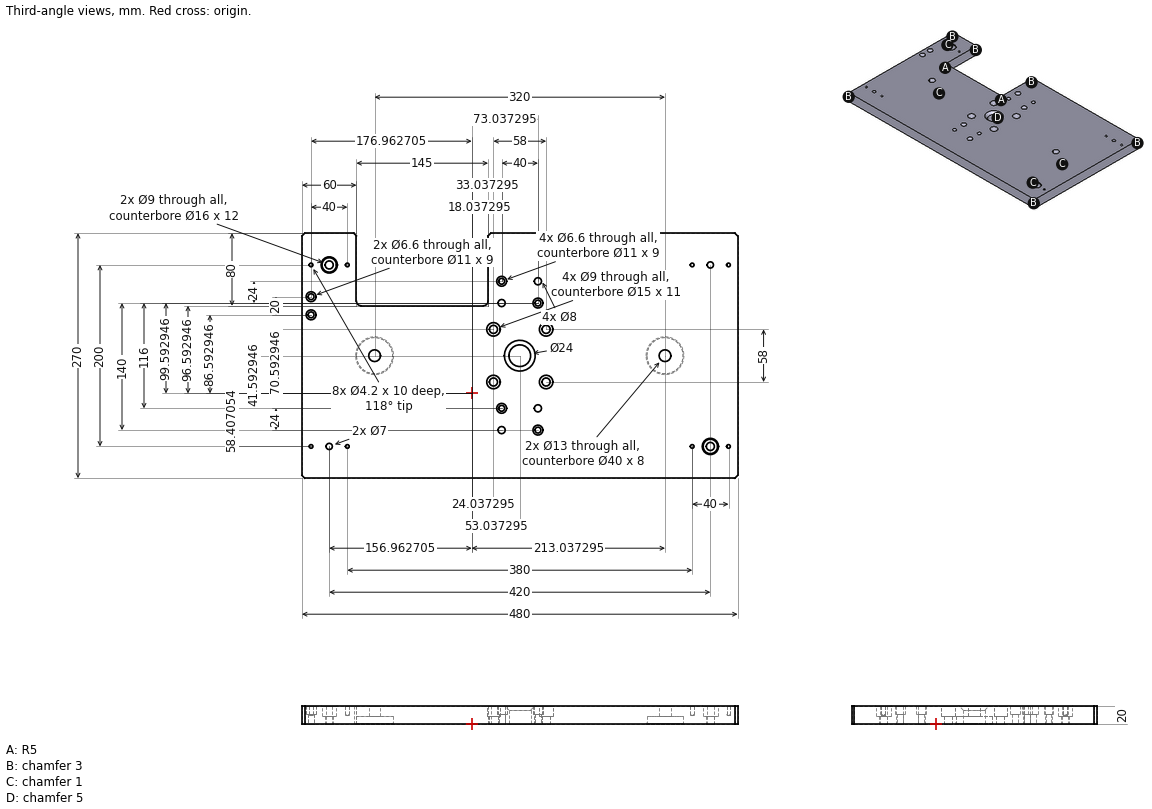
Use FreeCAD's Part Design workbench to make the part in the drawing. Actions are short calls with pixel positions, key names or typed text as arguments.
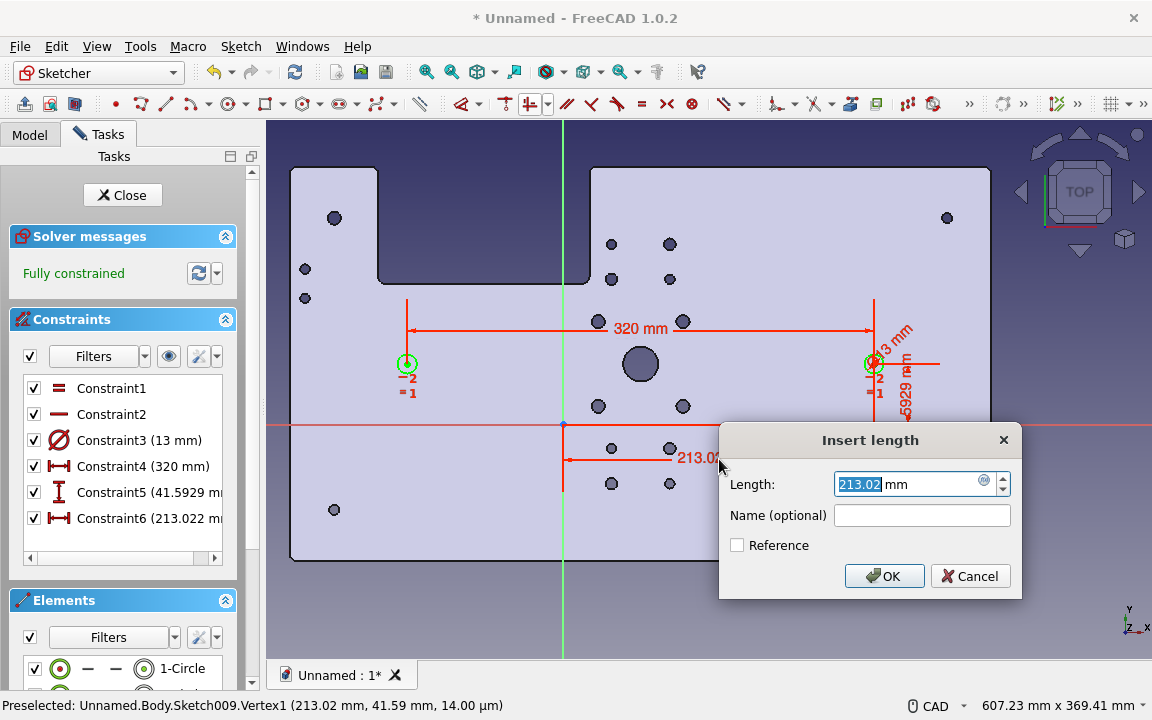
text(213.037295)
key(Return)
key(Escape)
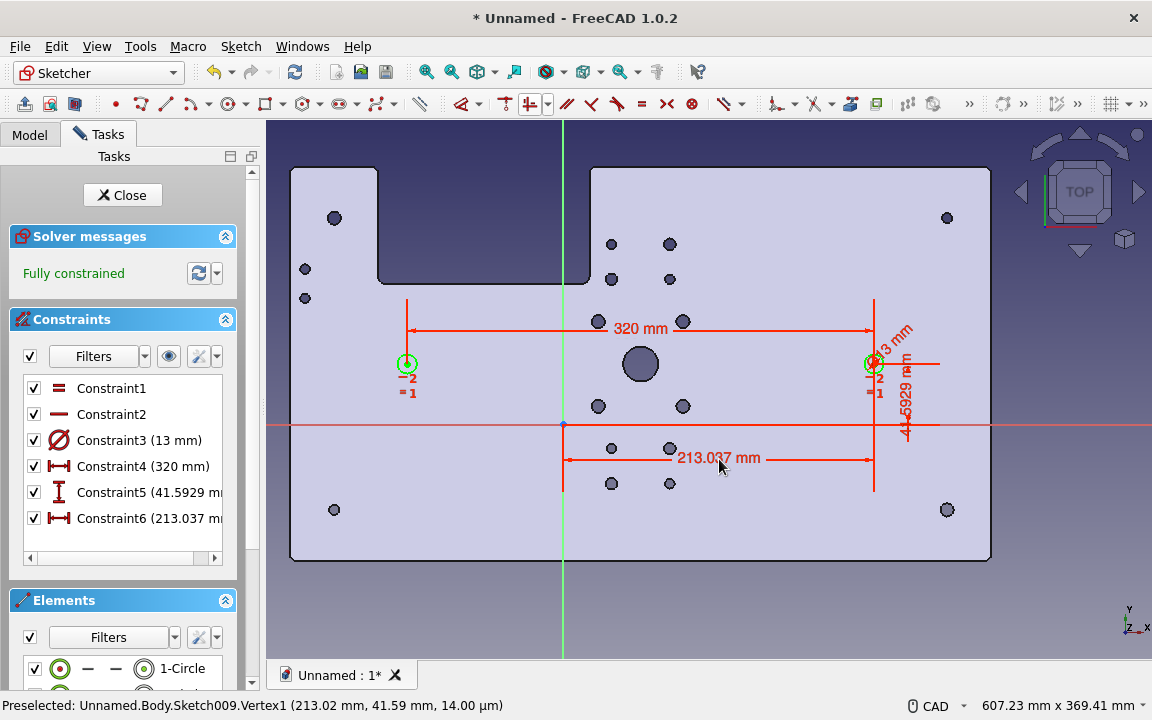
click(123, 195)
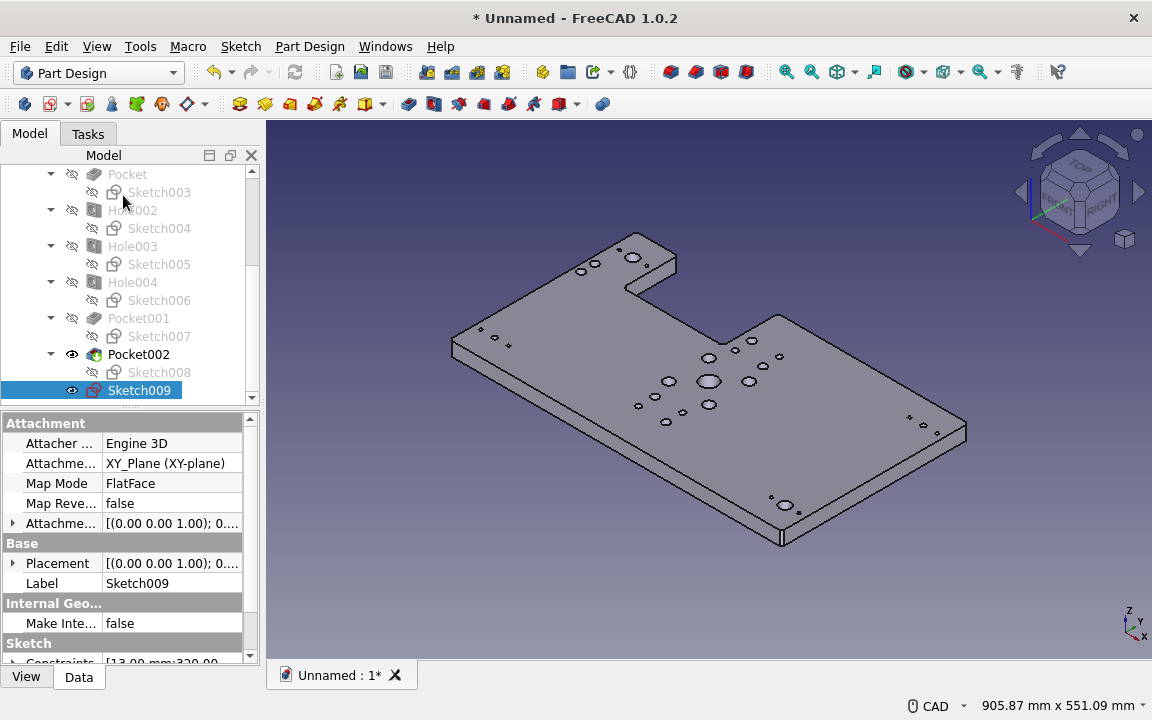
click(434, 104)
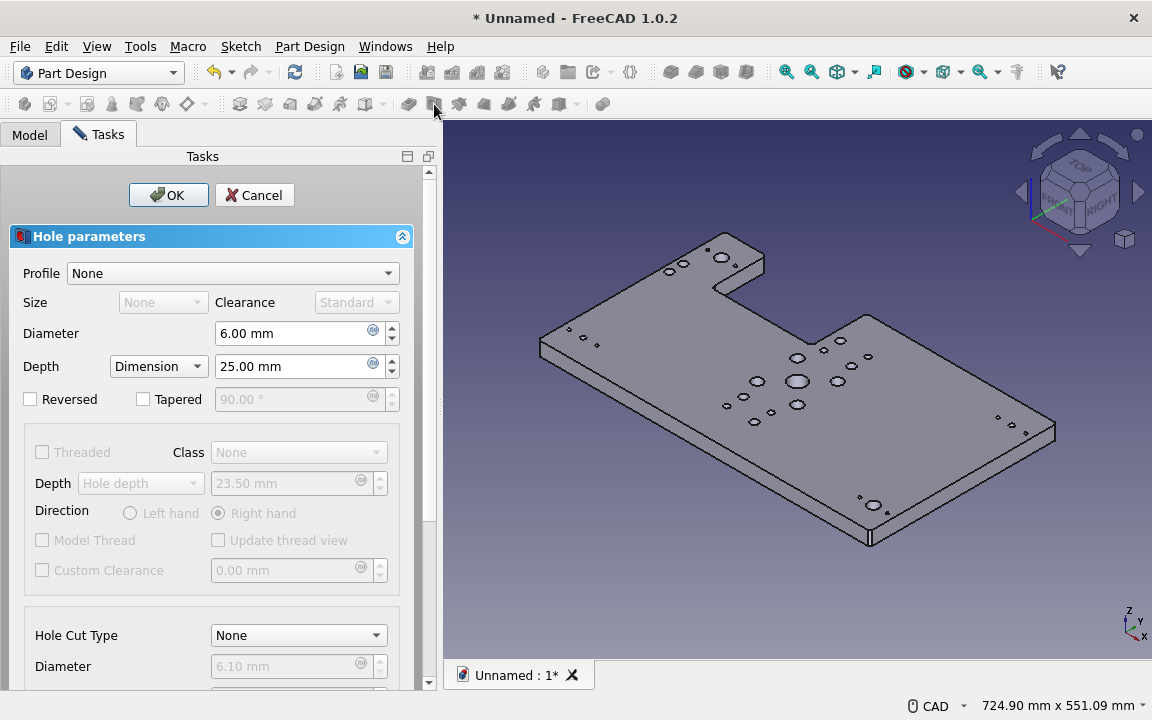
triple_click(300, 334)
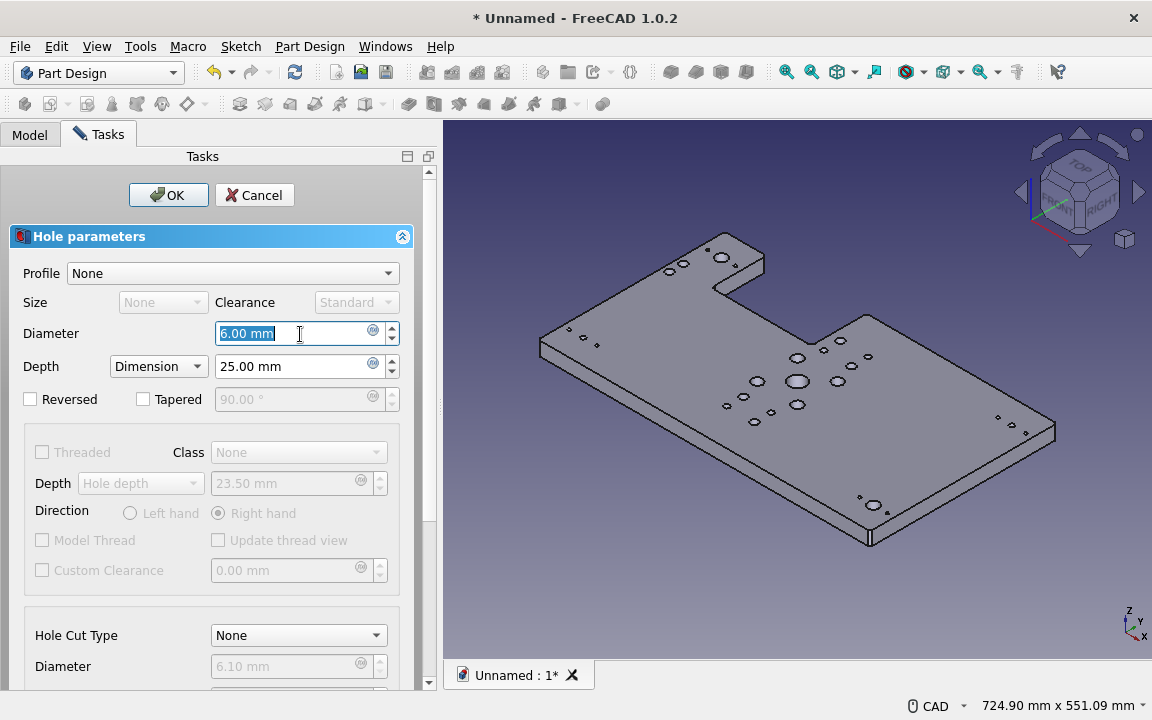
text(13)
key(Tab)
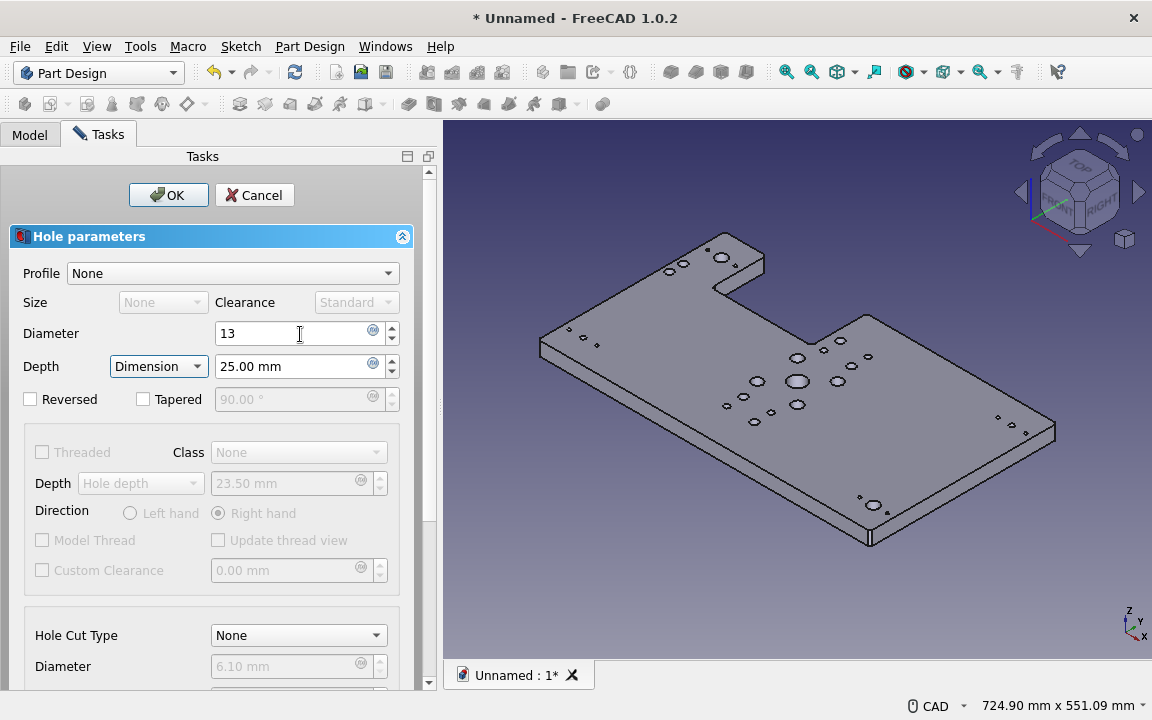
click(160, 366)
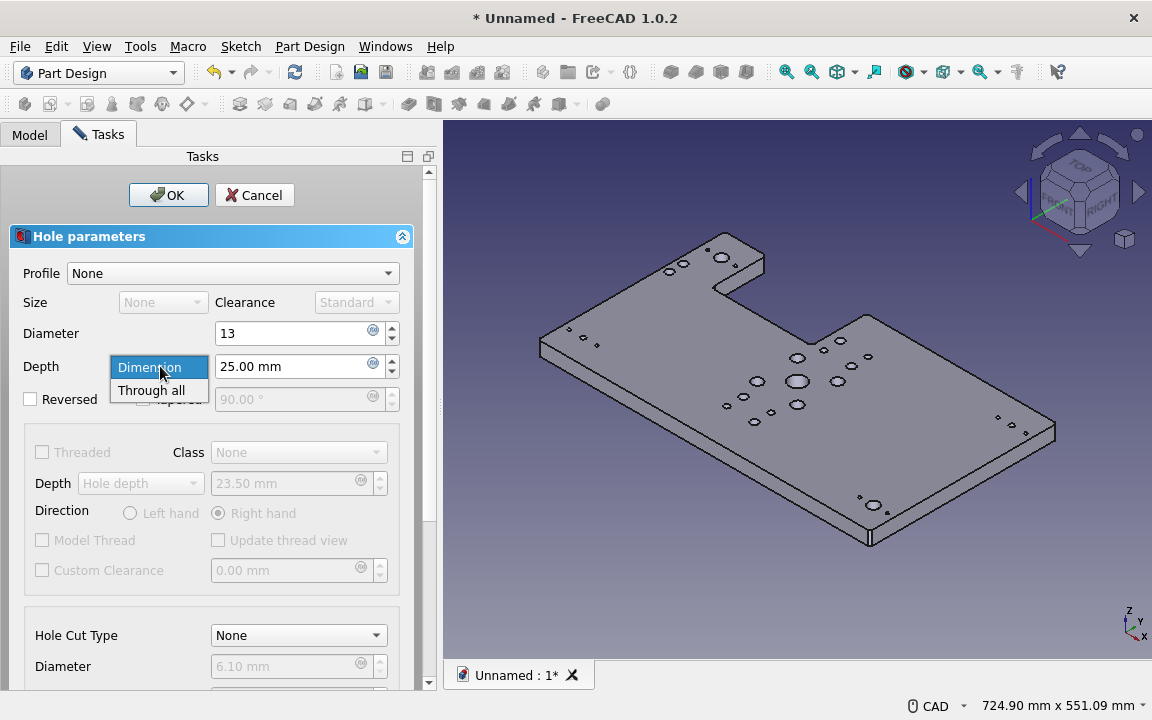
click(158, 390)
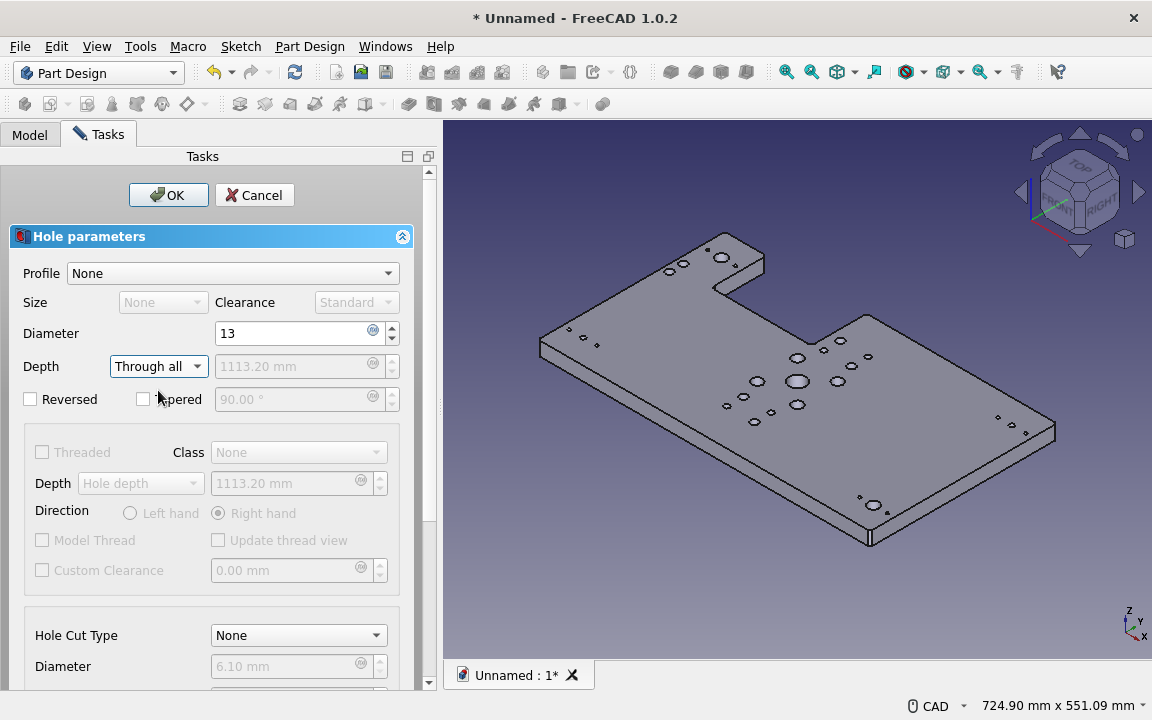
click(31, 399)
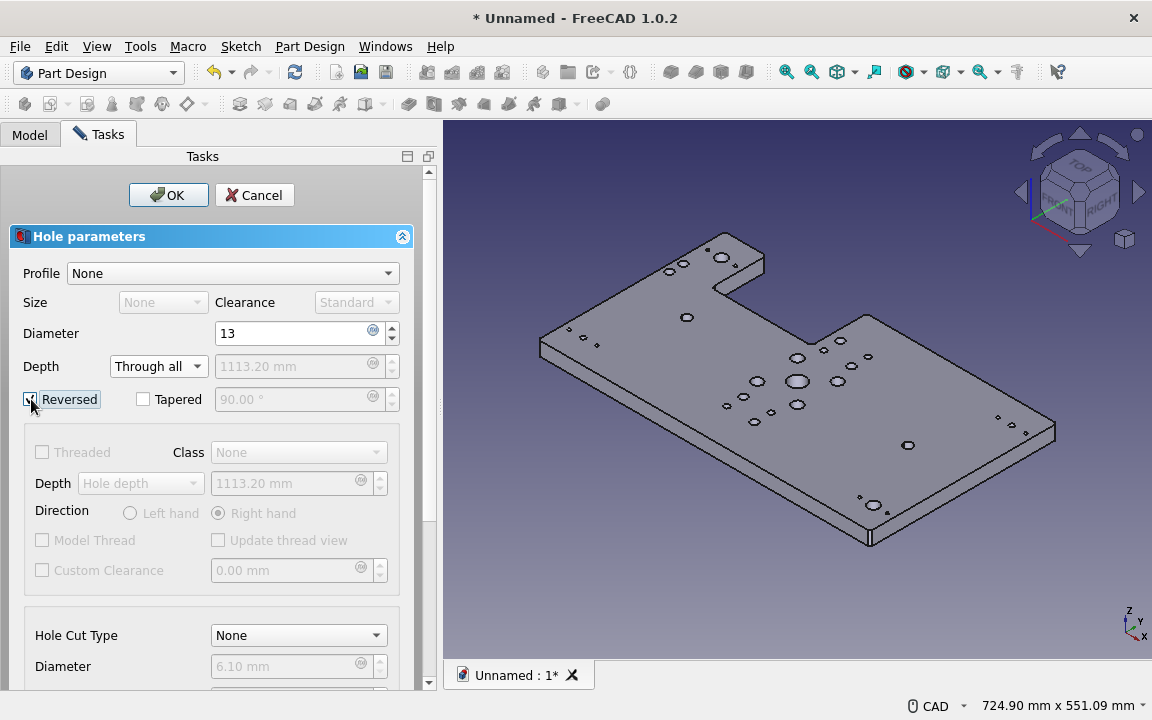
click(300, 636)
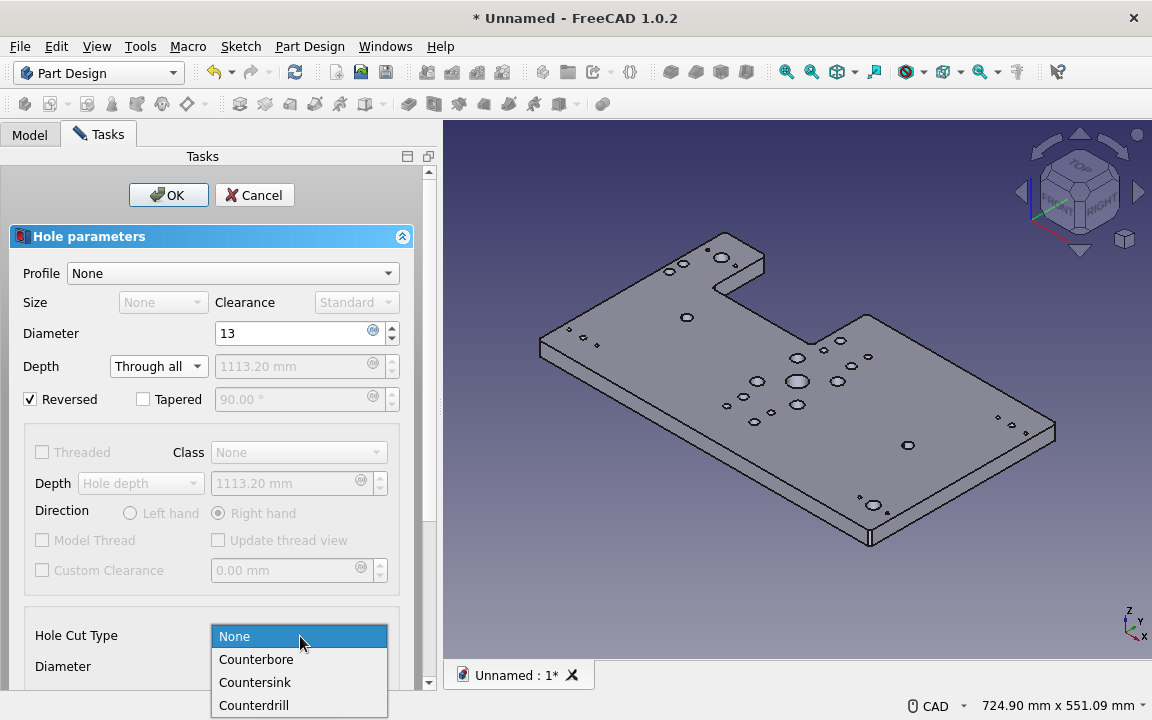
click(298, 660)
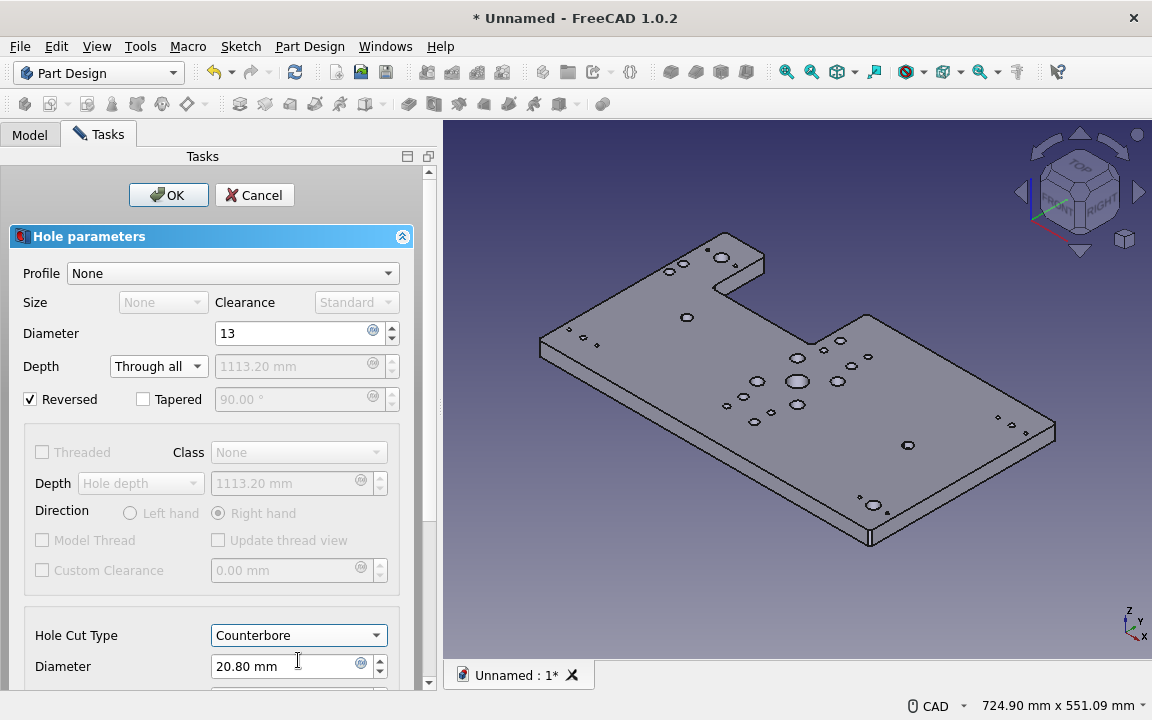
triple_click(292, 666)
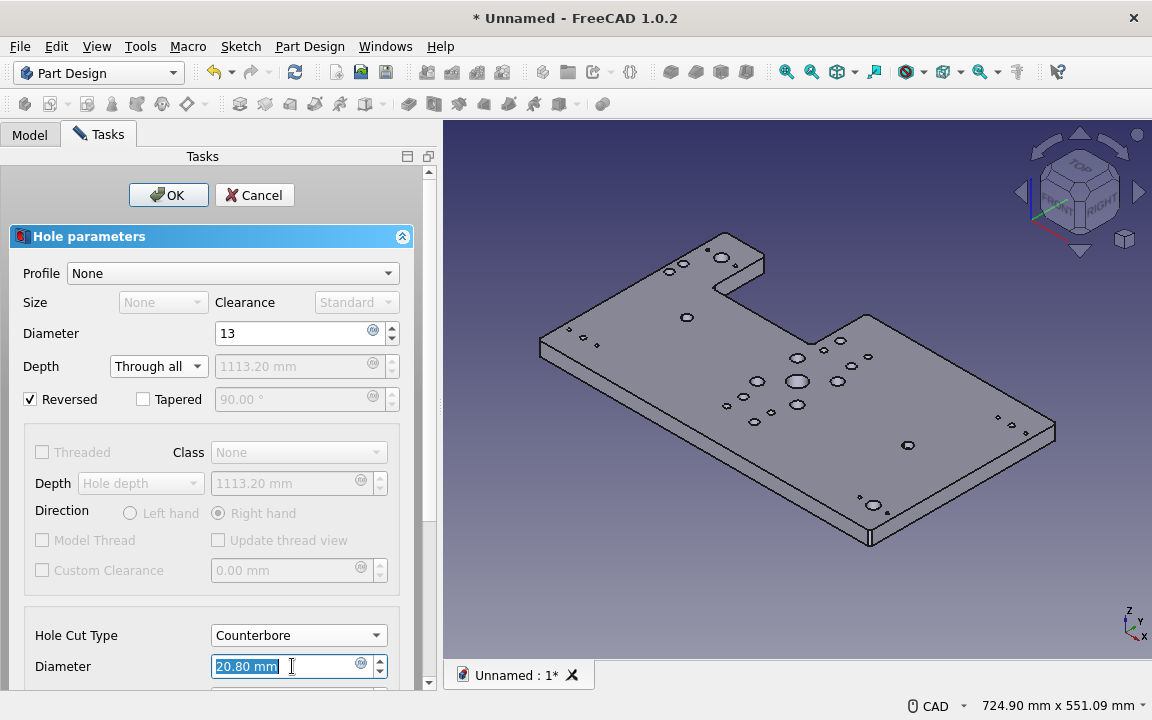
text(40)
key(Tab)